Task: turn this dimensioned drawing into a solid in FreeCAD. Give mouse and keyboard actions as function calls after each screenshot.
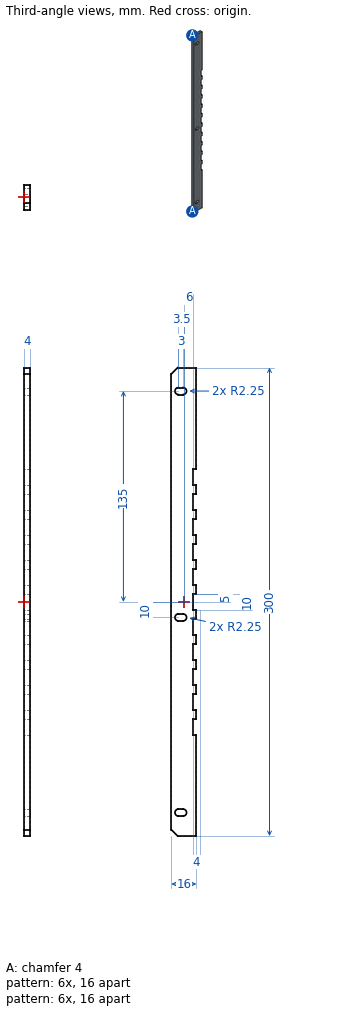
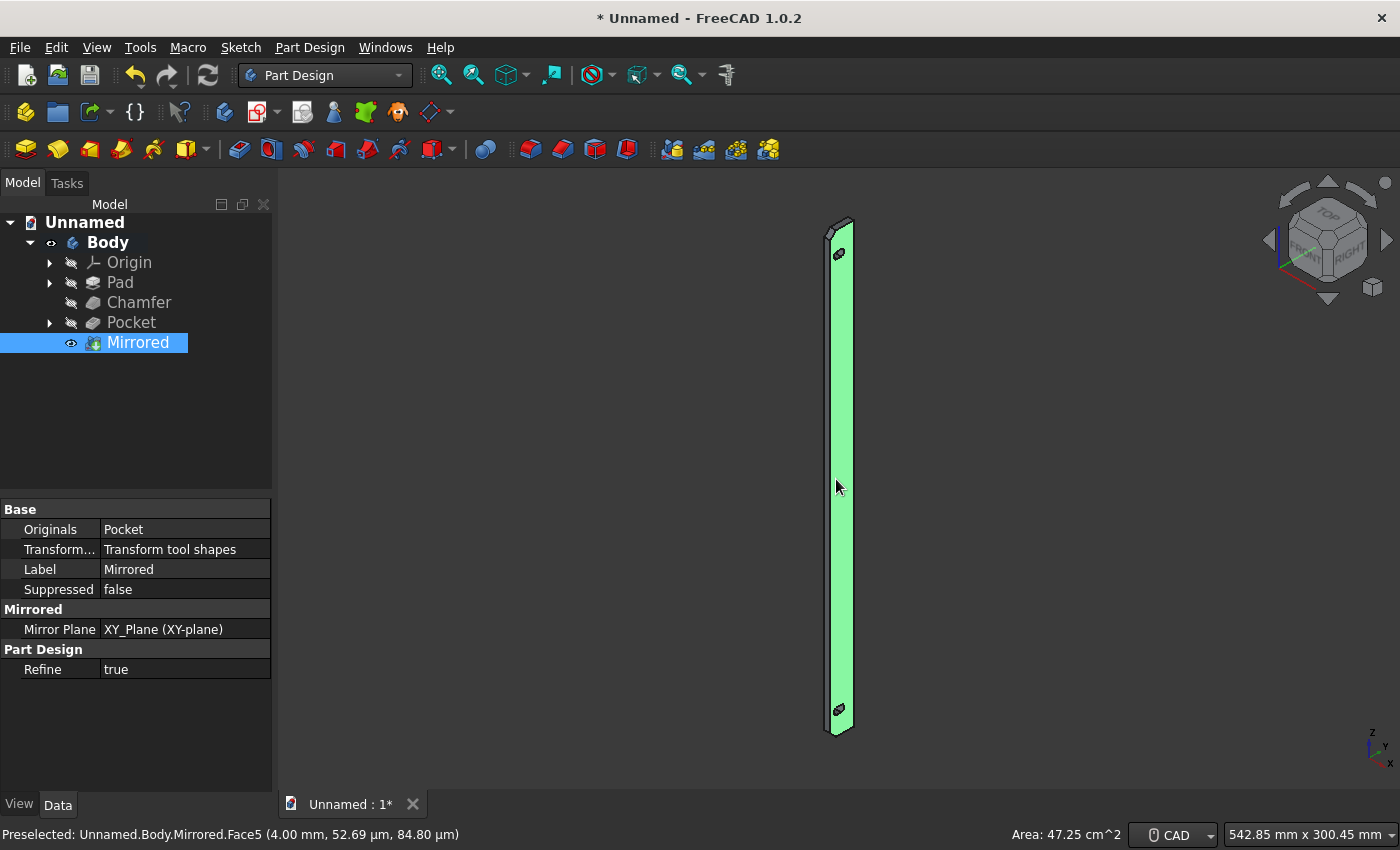
click(258, 112)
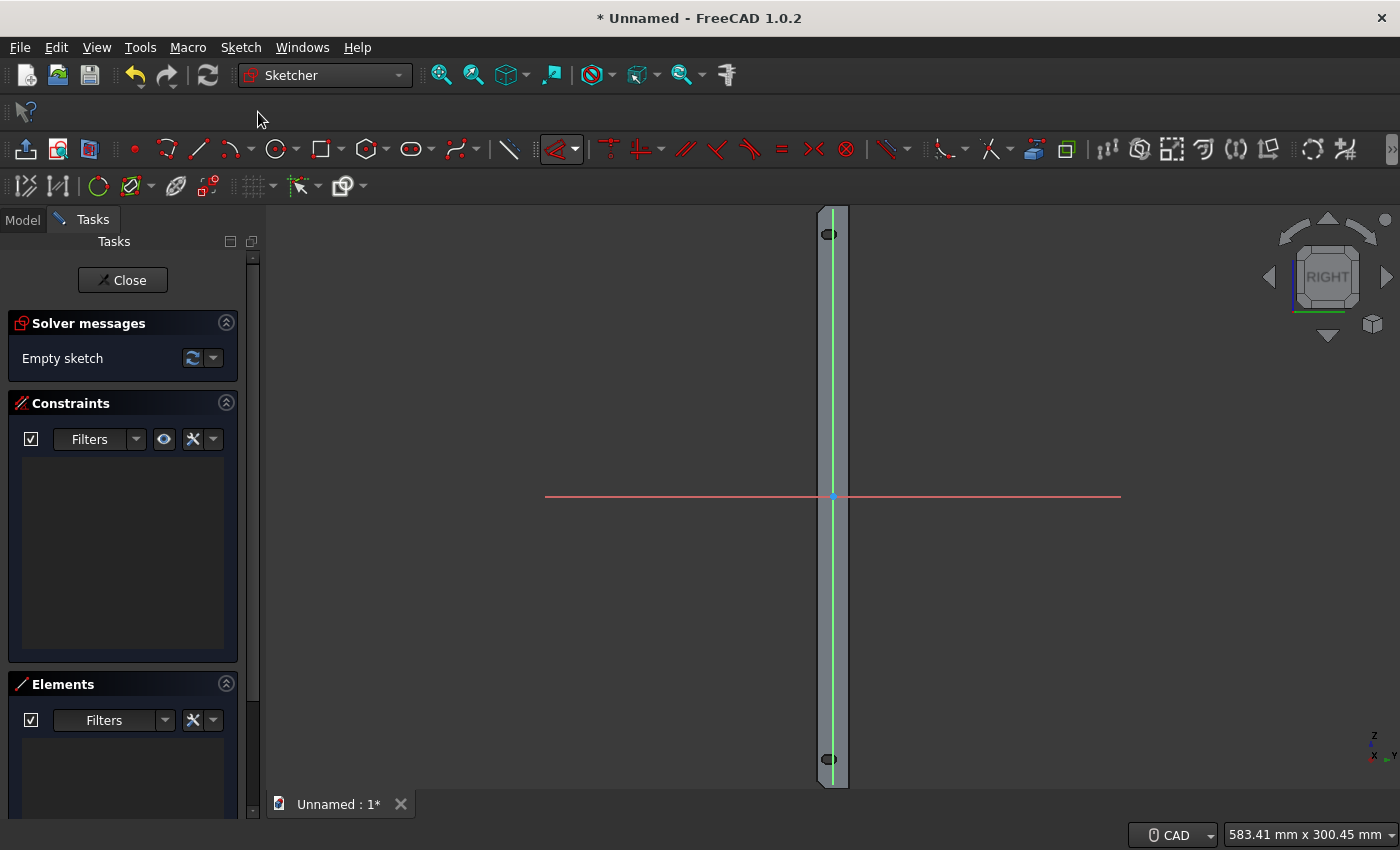
scroll(847, 497, up, 15)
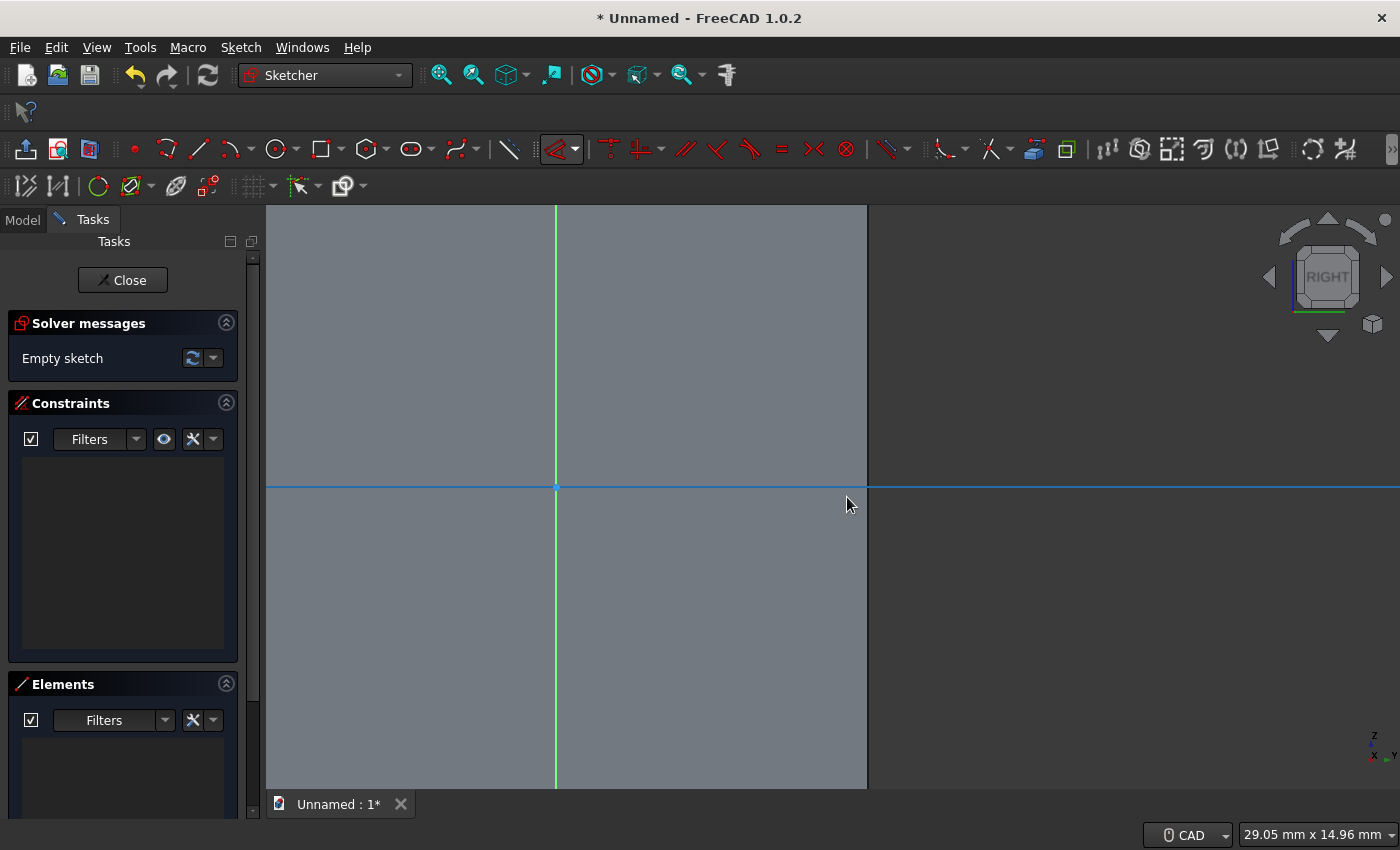
key(g)
key(r)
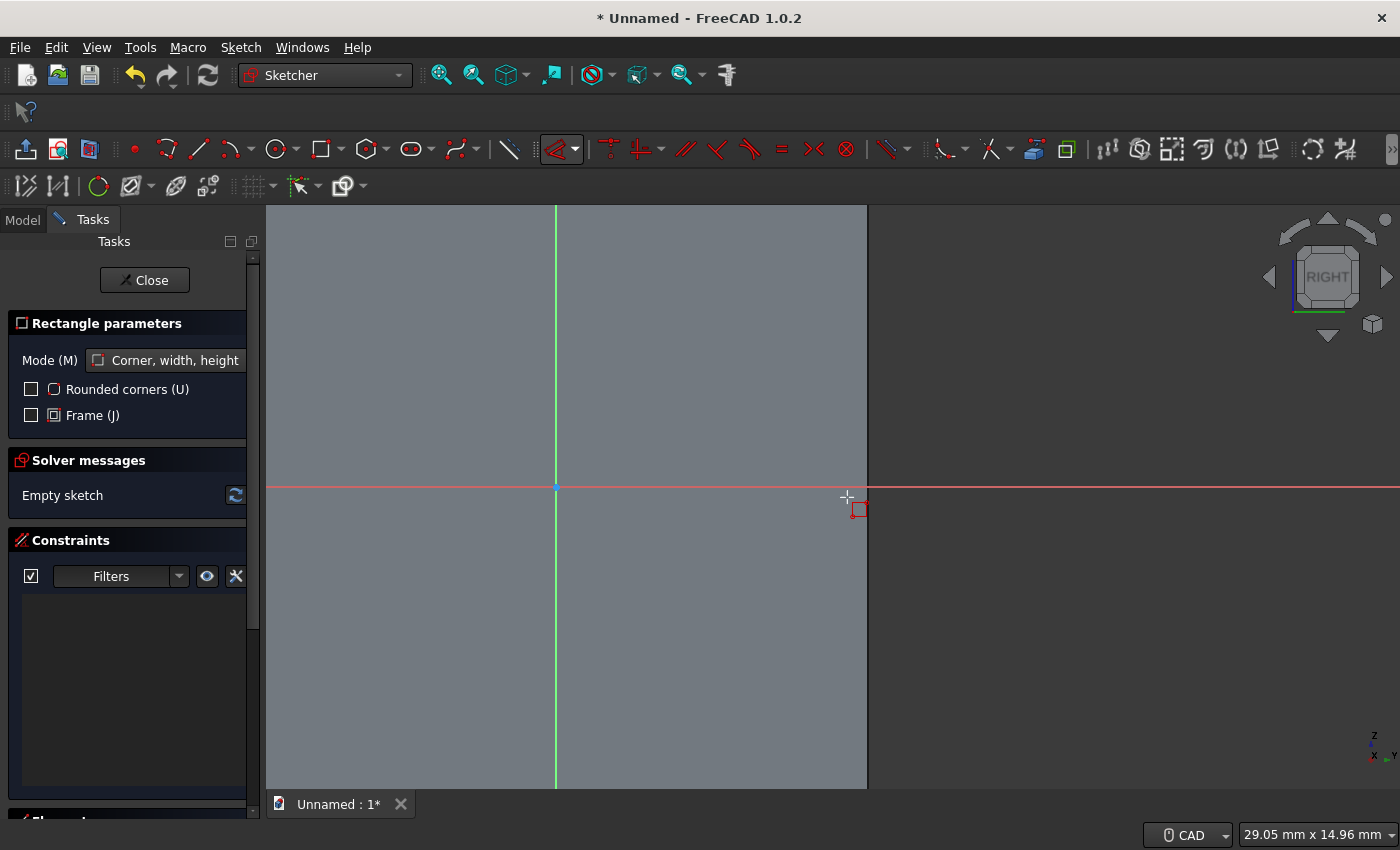
click(790, 292)
click(946, 683)
key(Escape)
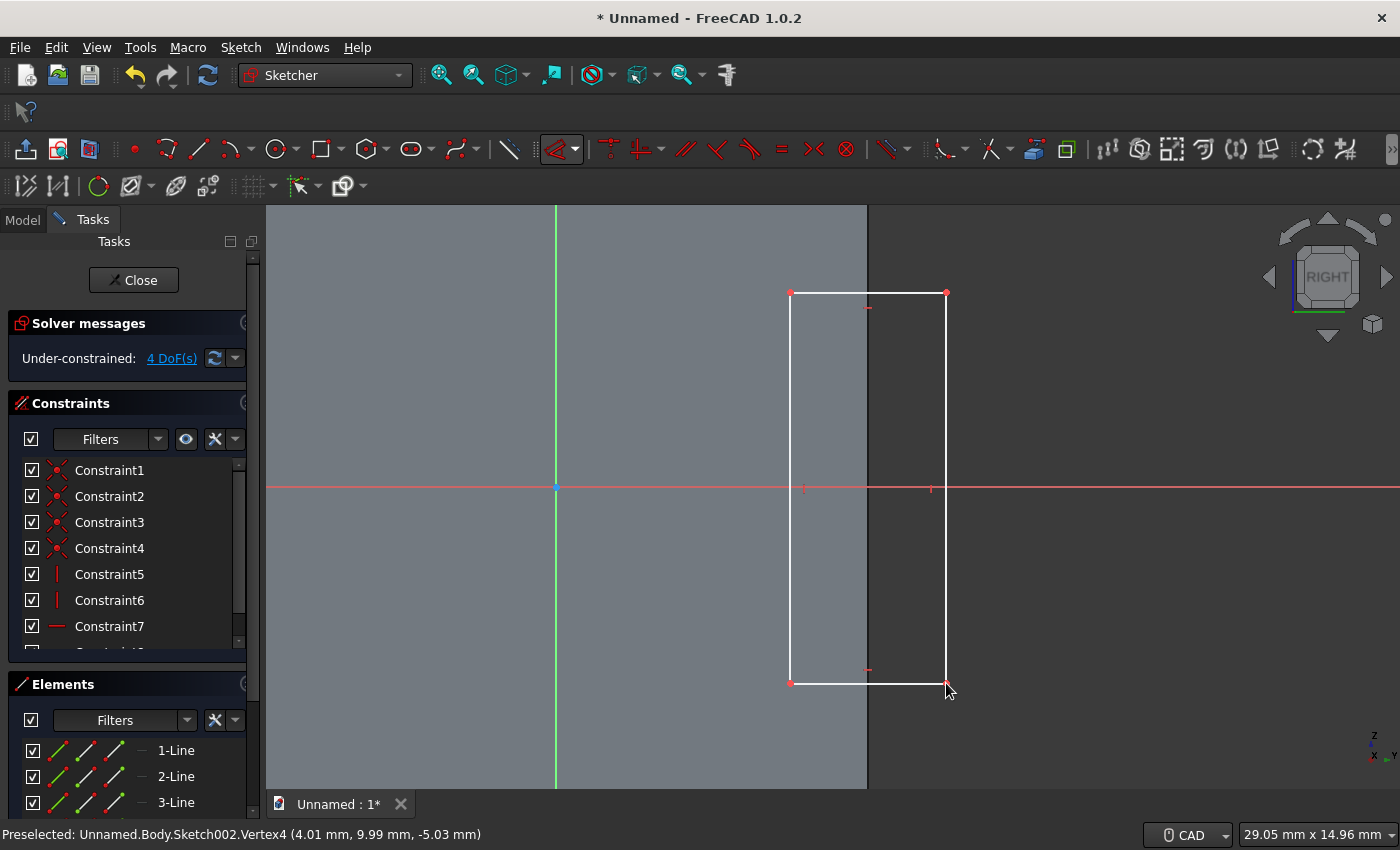
click(837, 684)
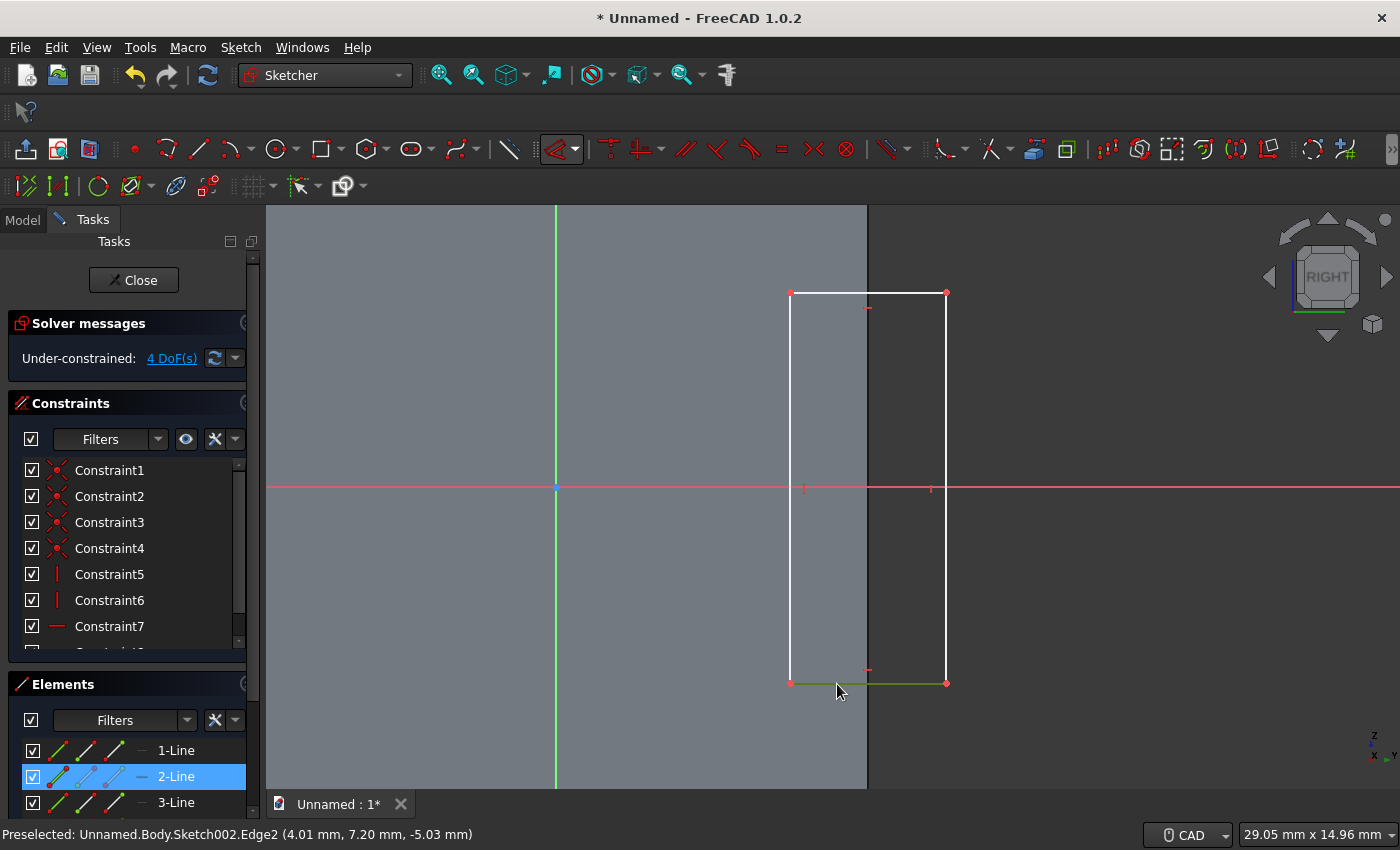
key(l)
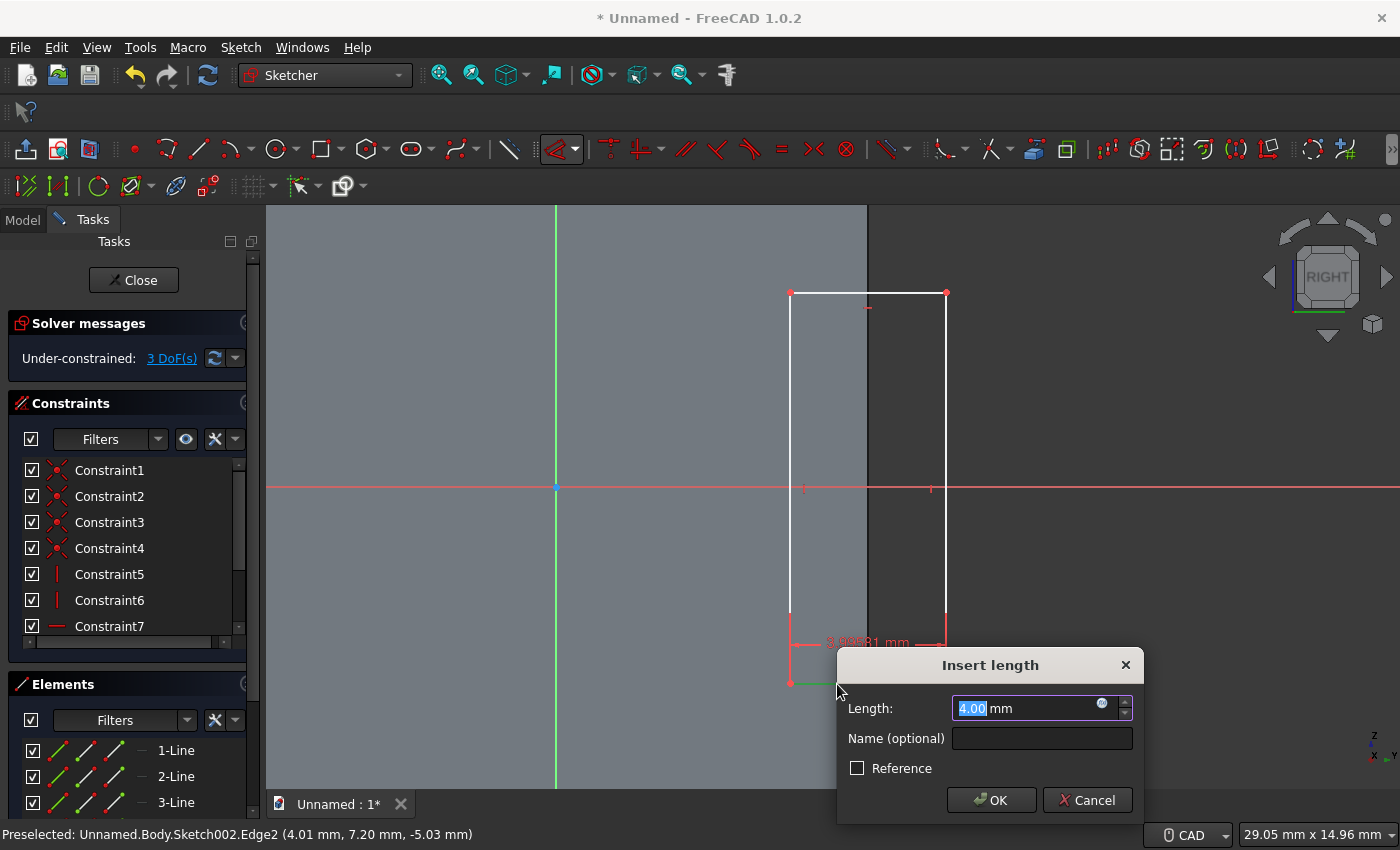
text(4)
key(Return)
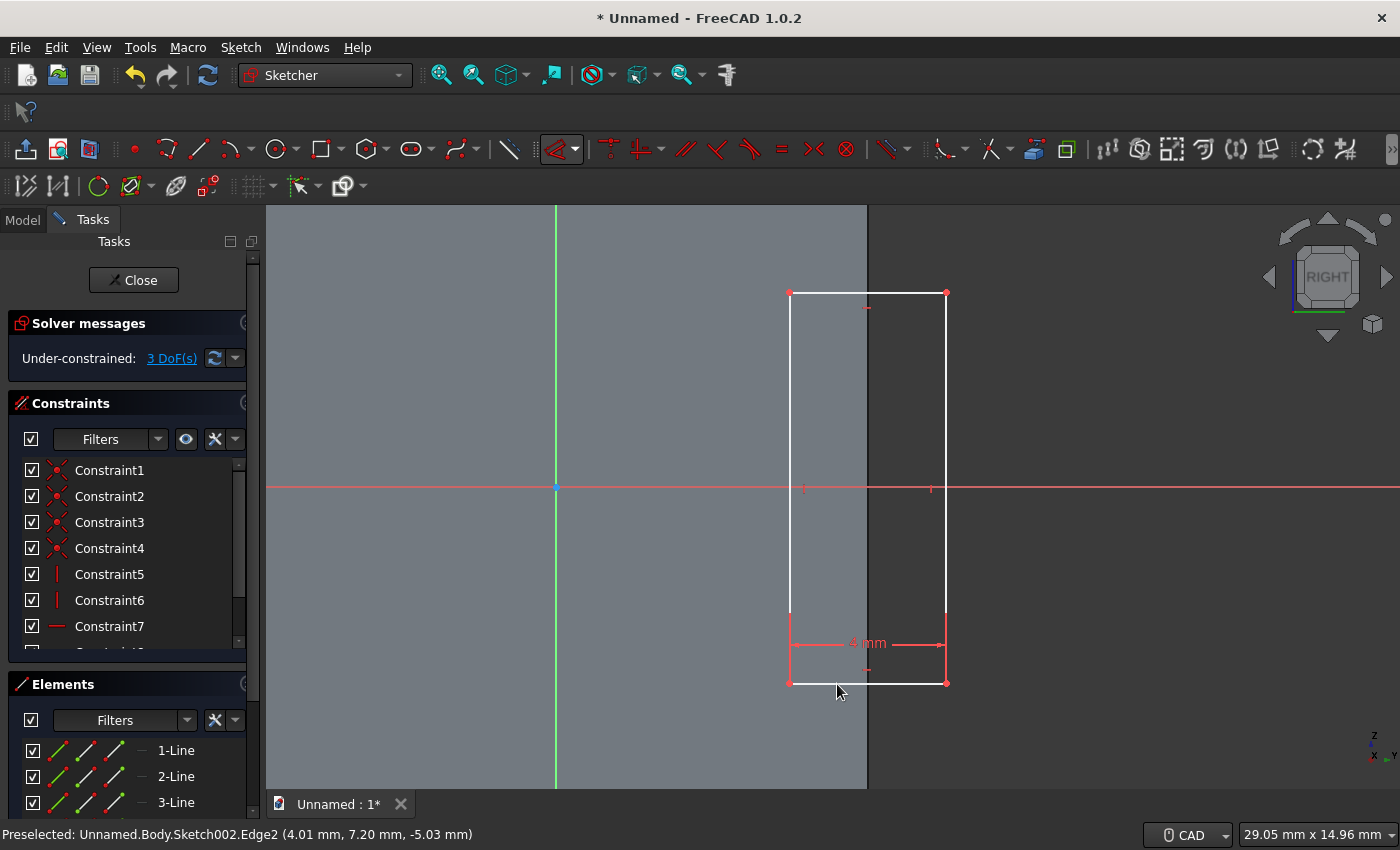
click(790, 410)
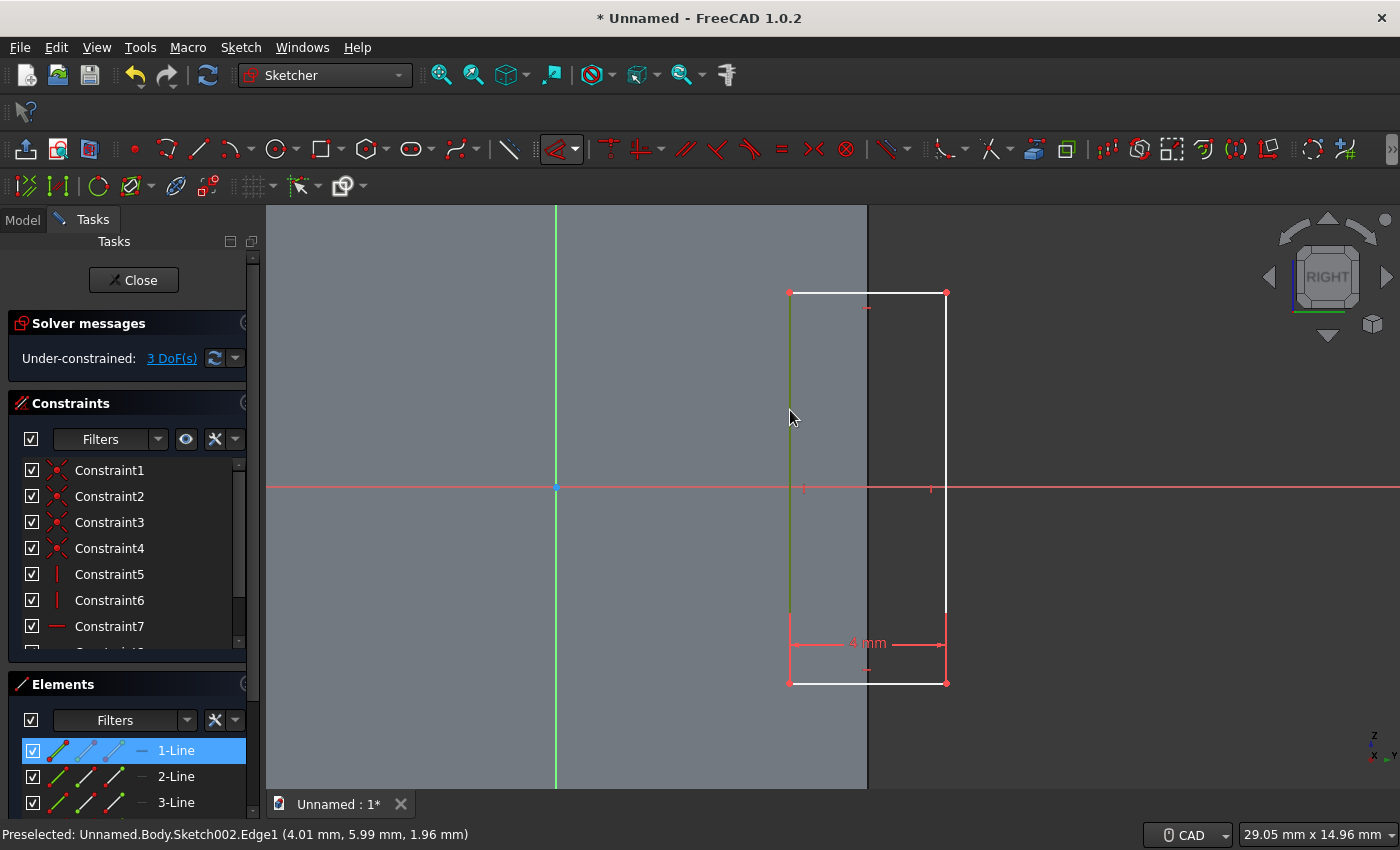
key(i)